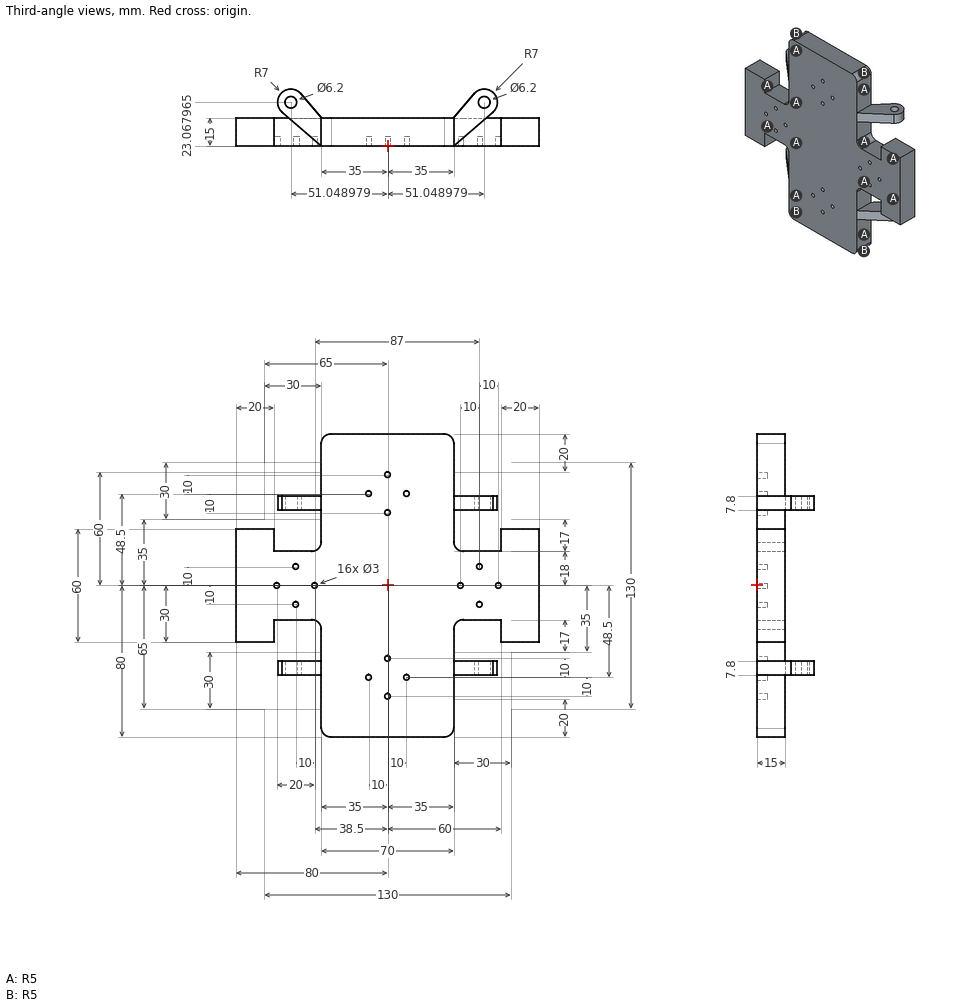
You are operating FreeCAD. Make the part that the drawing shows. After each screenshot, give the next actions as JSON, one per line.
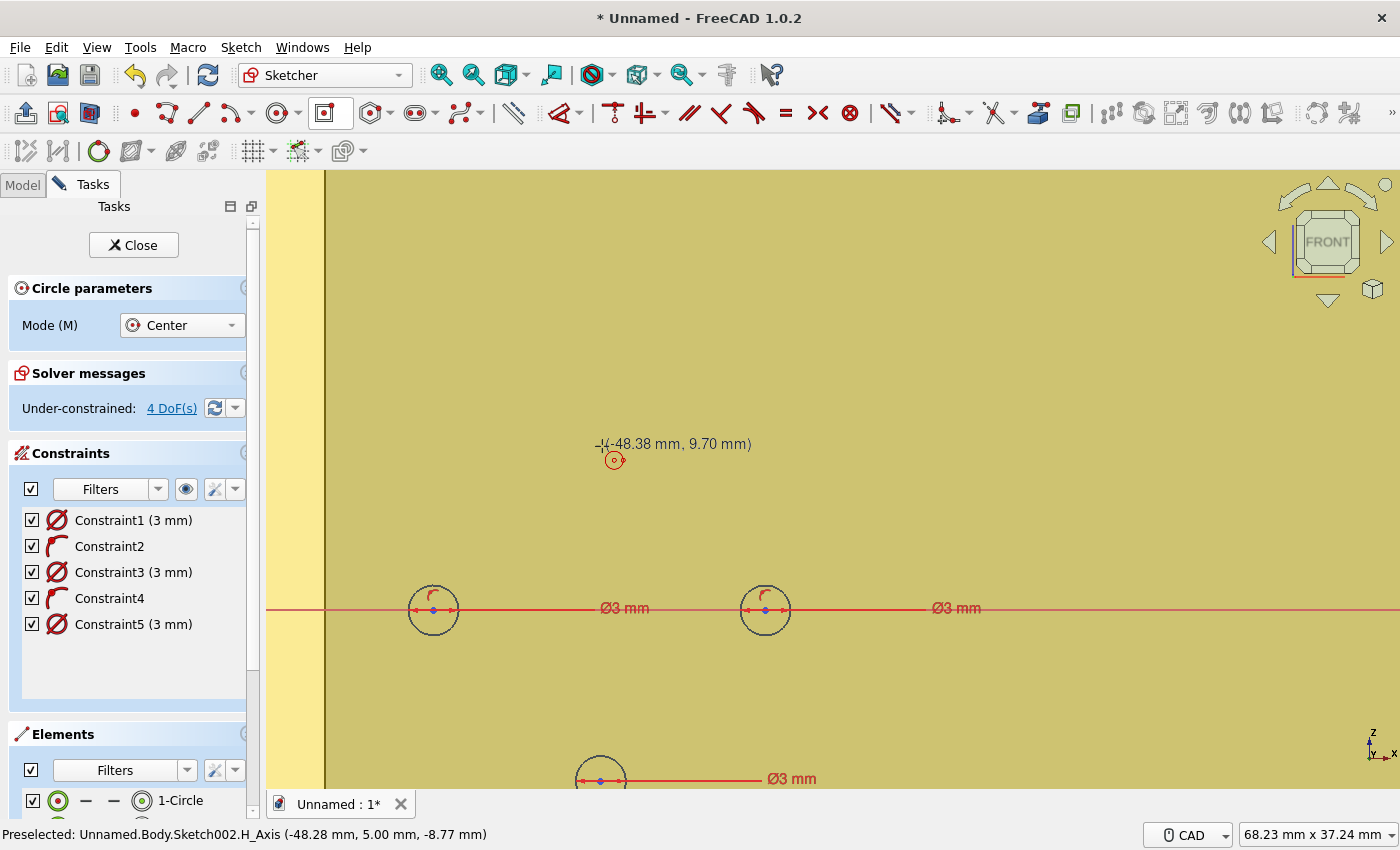
{"action": "scroll", "coordinate": [602, 446], "scroll_direction": "down", "scroll_amount": 8}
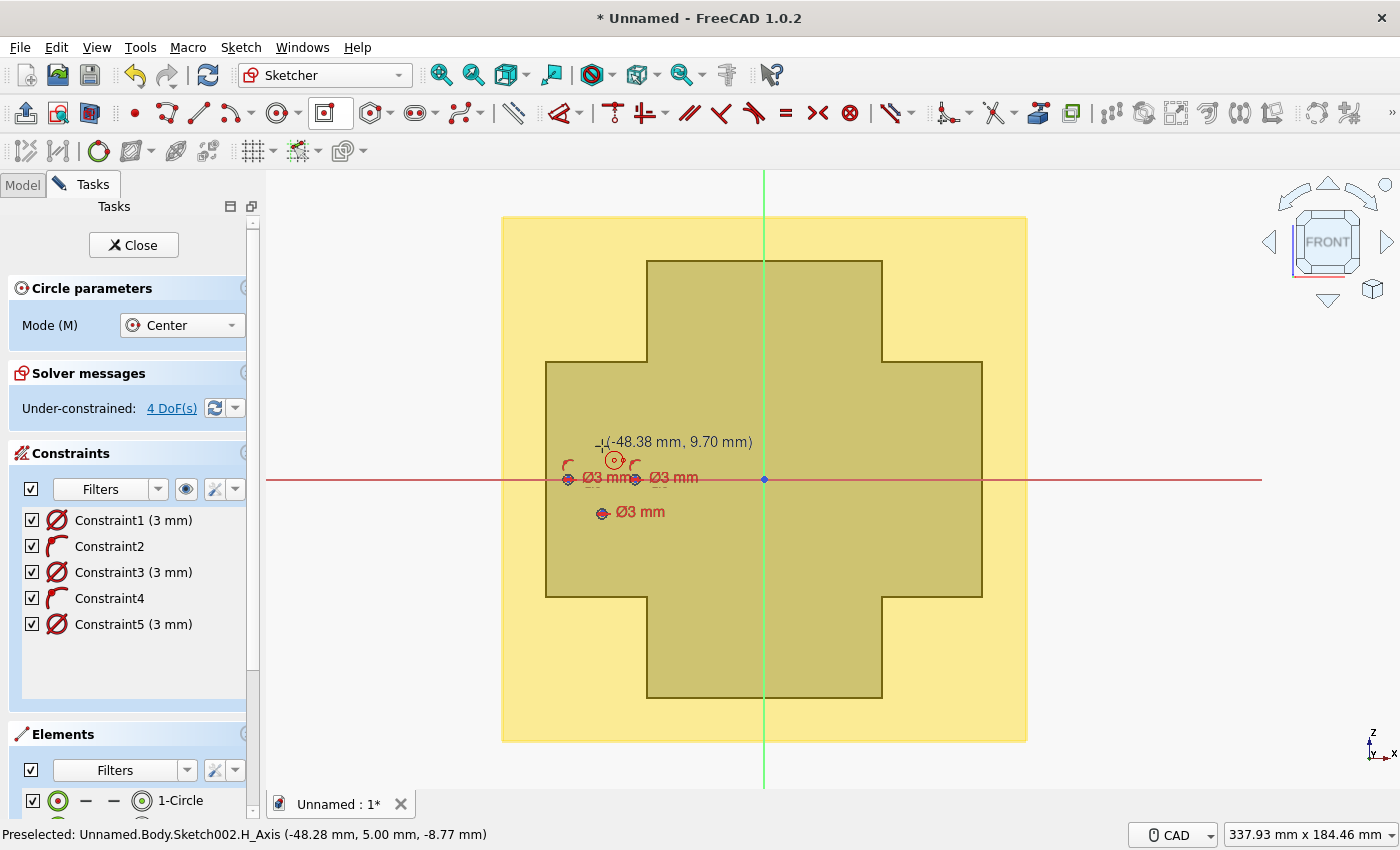
{"action": "left_click", "coordinate": [602, 446]}
{"action": "mouse_move", "coordinate": [605, 442]}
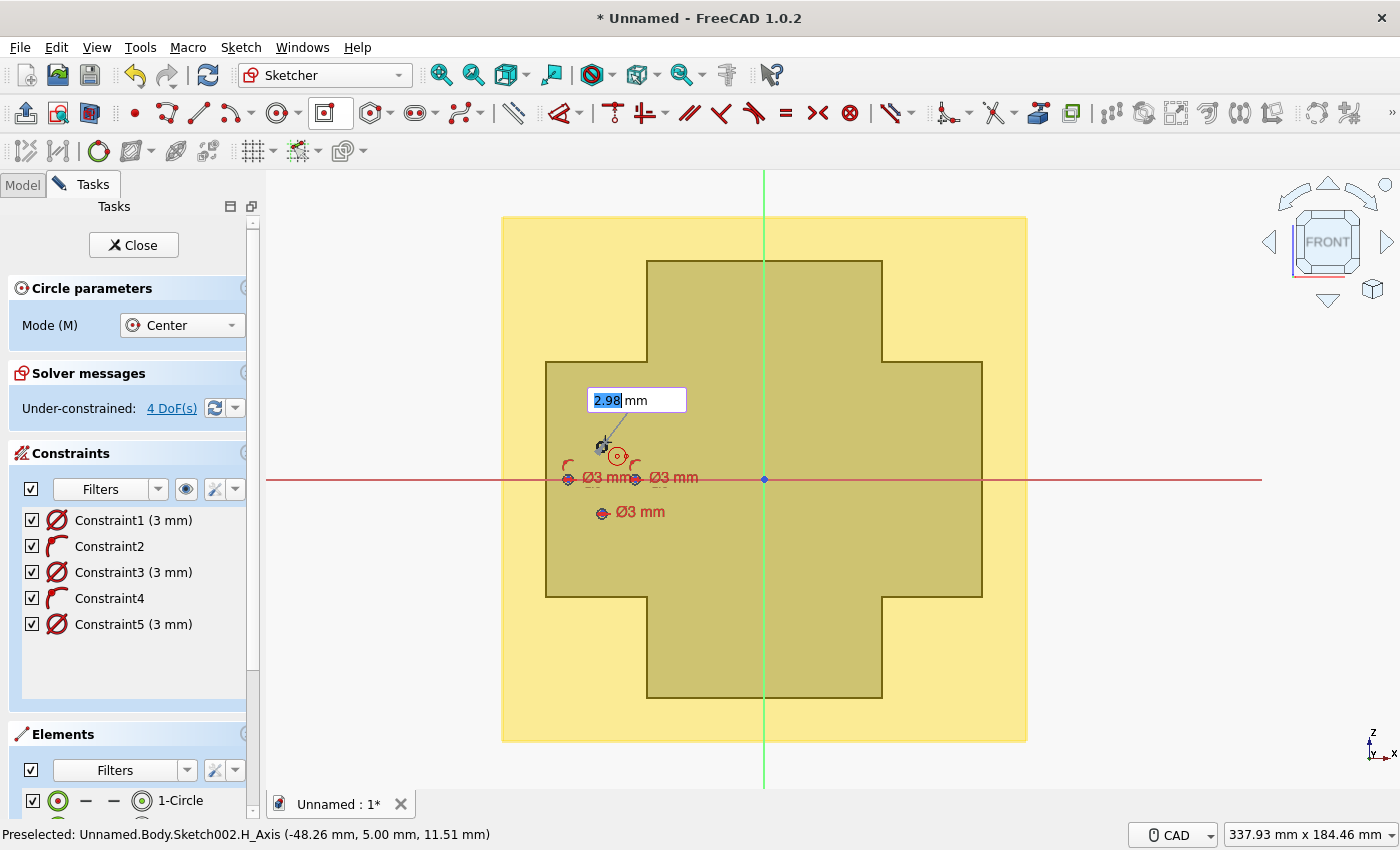
{"action": "type", "text": "3"}
{"action": "key", "text": "Return"}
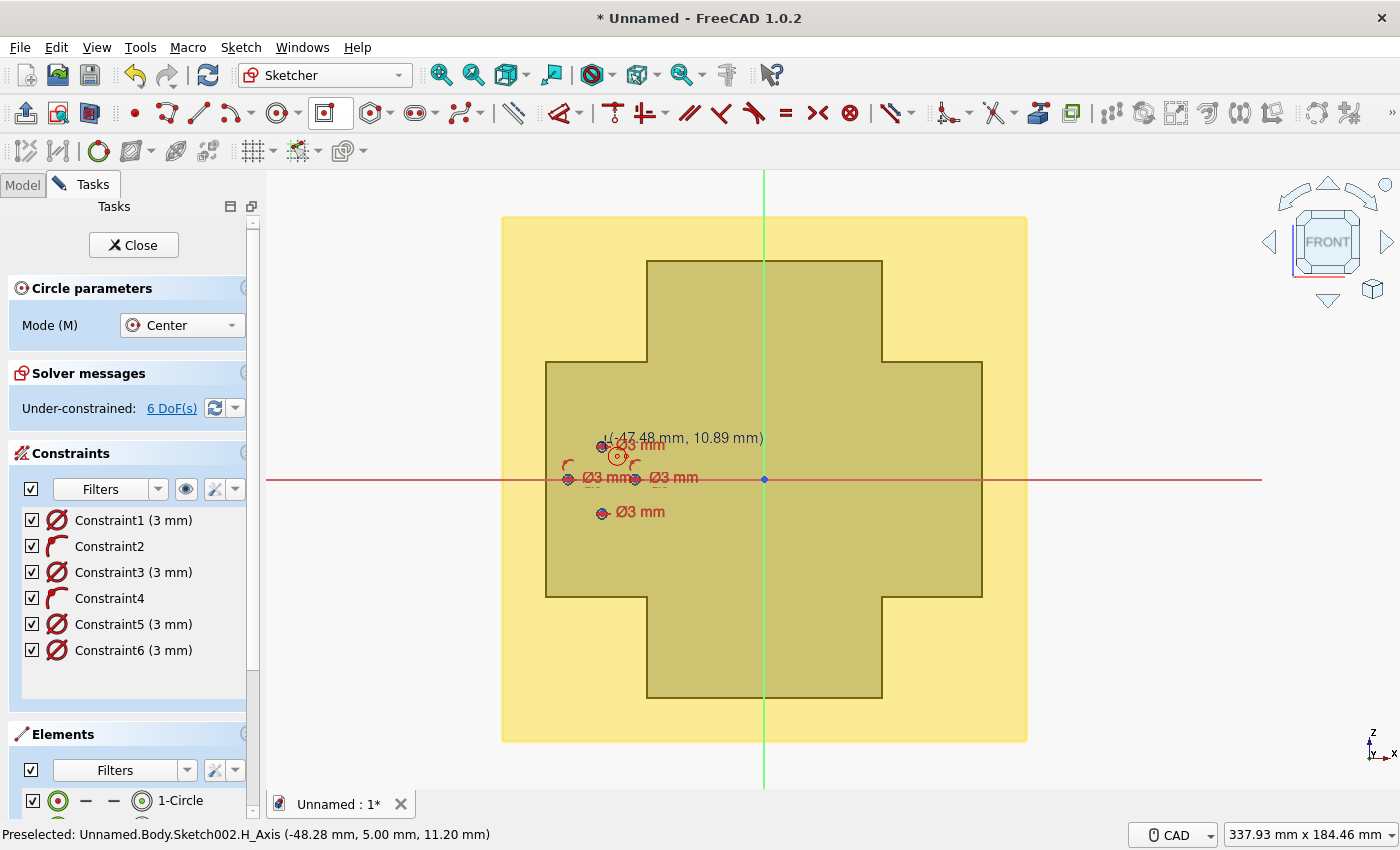
{"action": "scroll", "coordinate": [798, 642], "scroll_direction": "up", "scroll_amount": 8}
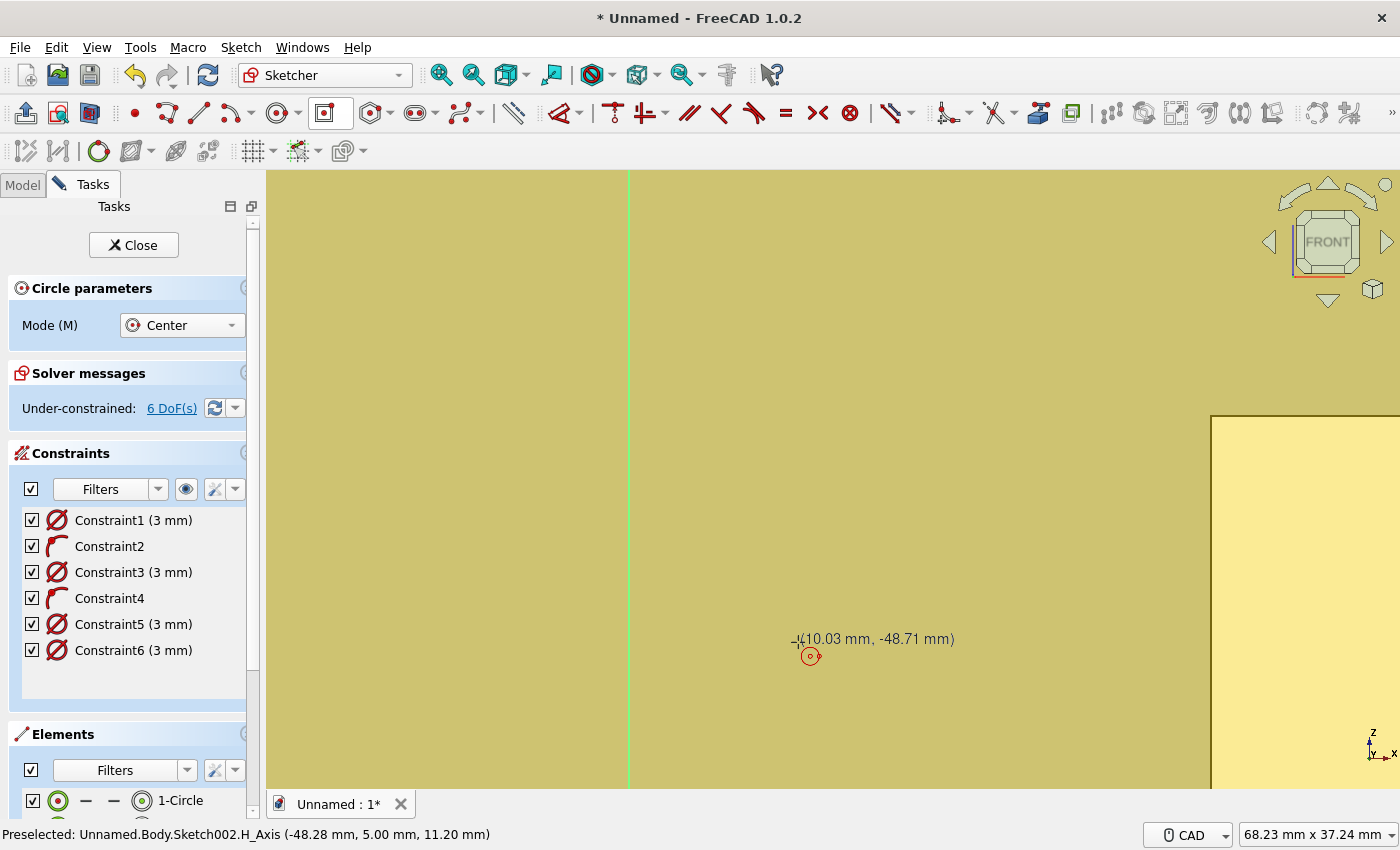
{"action": "scroll", "coordinate": [799, 643], "scroll_direction": "down", "scroll_amount": 8}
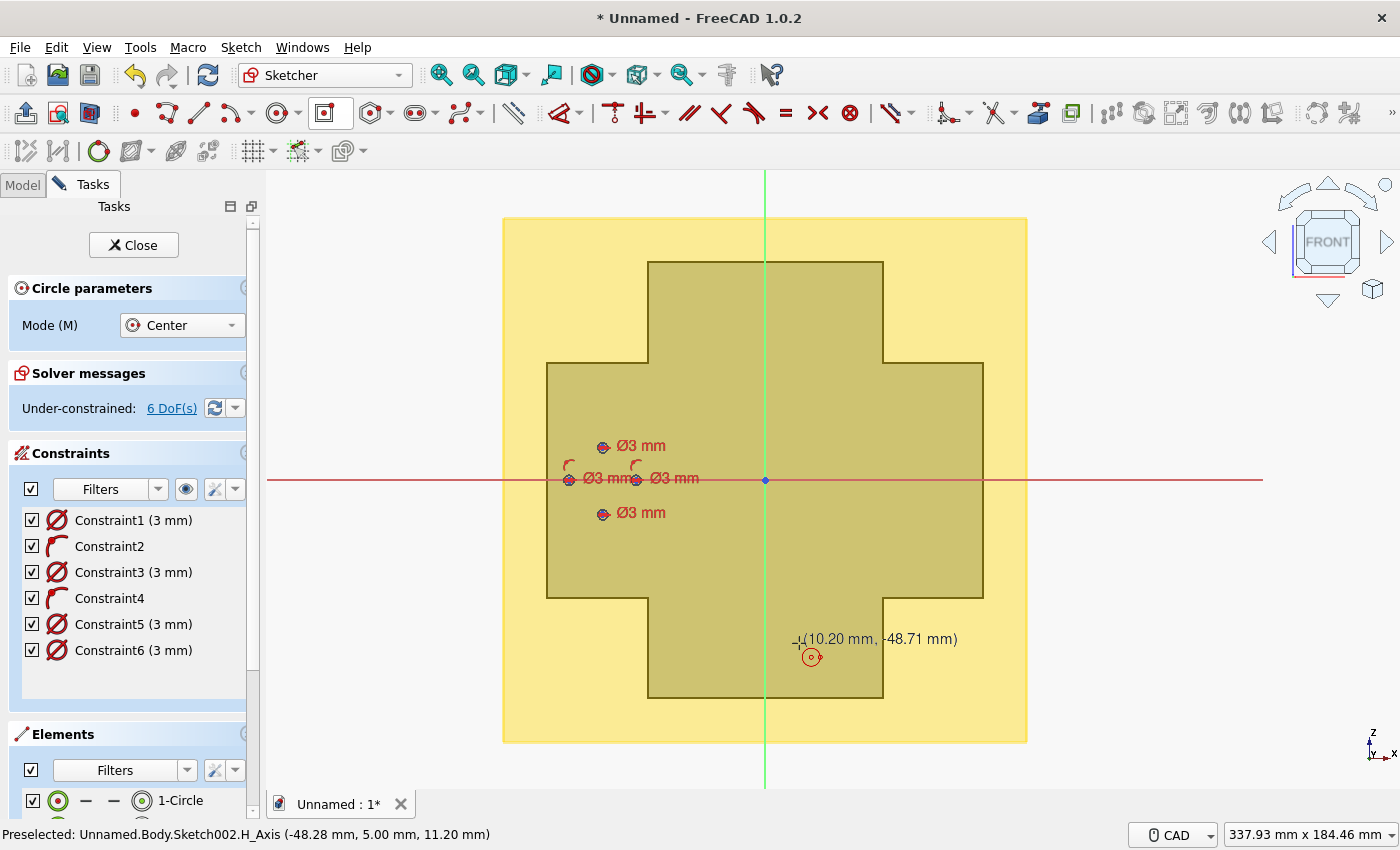
{"action": "left_click", "coordinate": [799, 643]}
{"action": "mouse_move", "coordinate": [802, 640]}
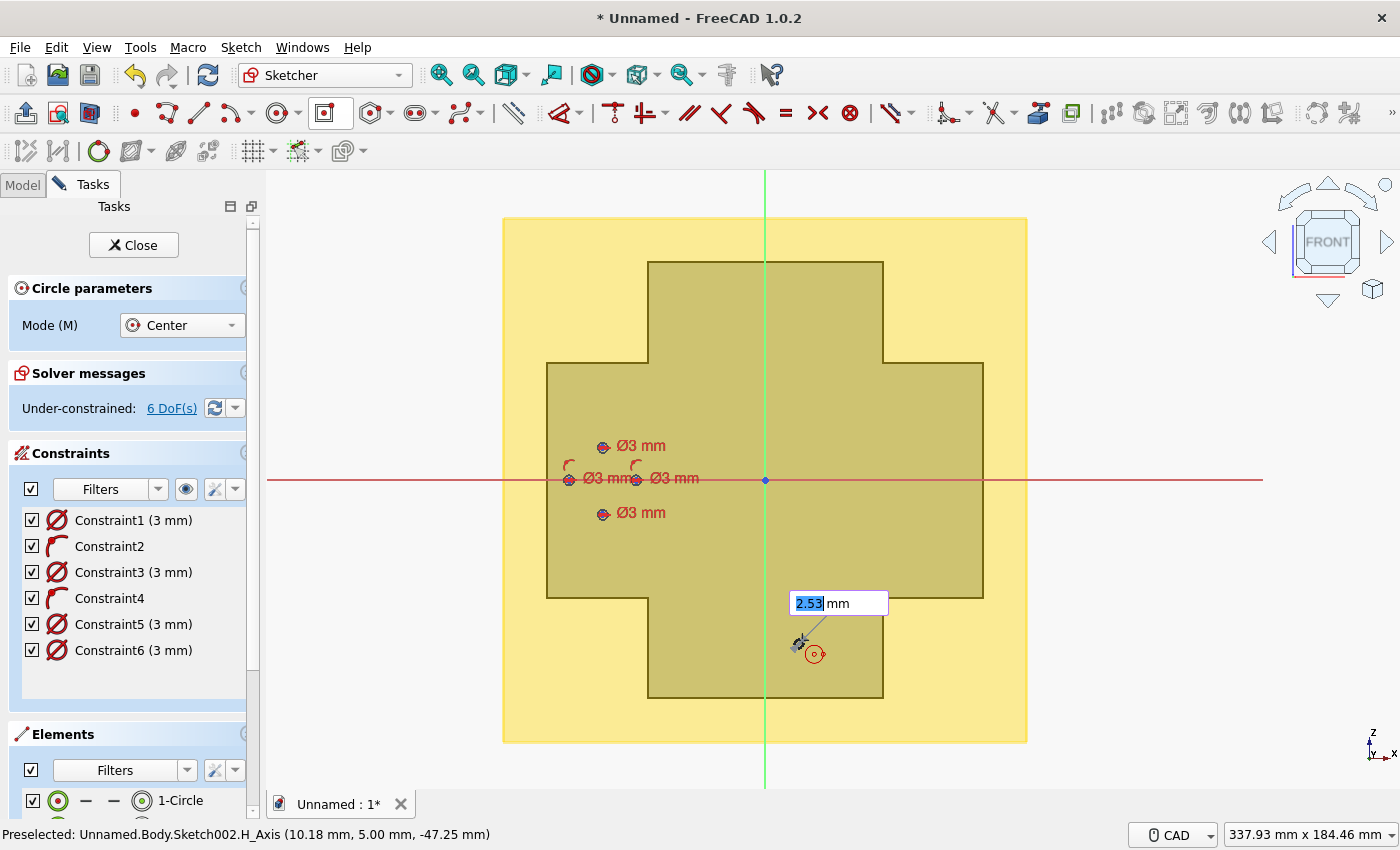
{"action": "type", "text": "3"}
{"action": "key", "text": "Return"}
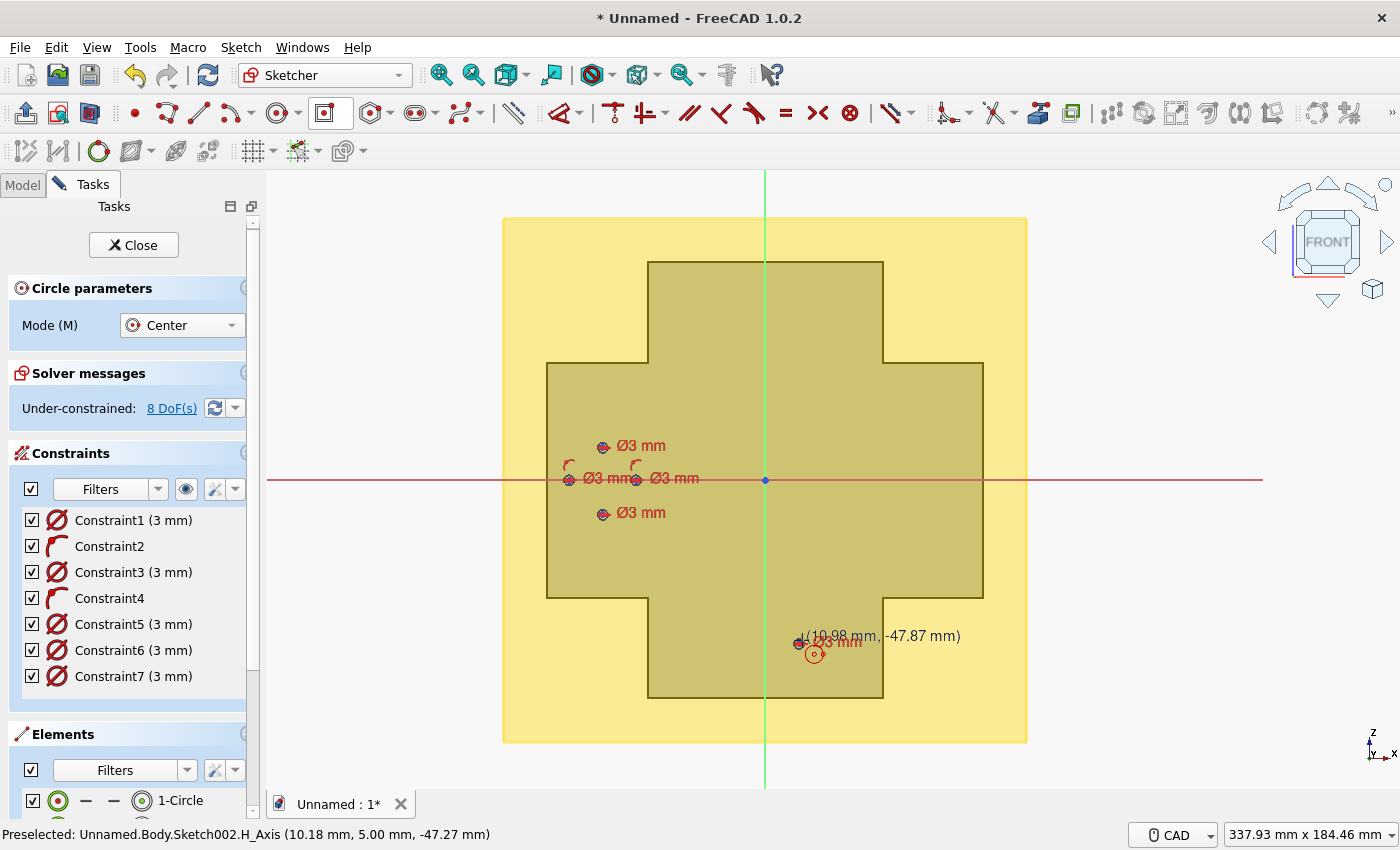
{"action": "scroll", "coordinate": [765, 610], "scroll_direction": "up", "scroll_amount": 8}